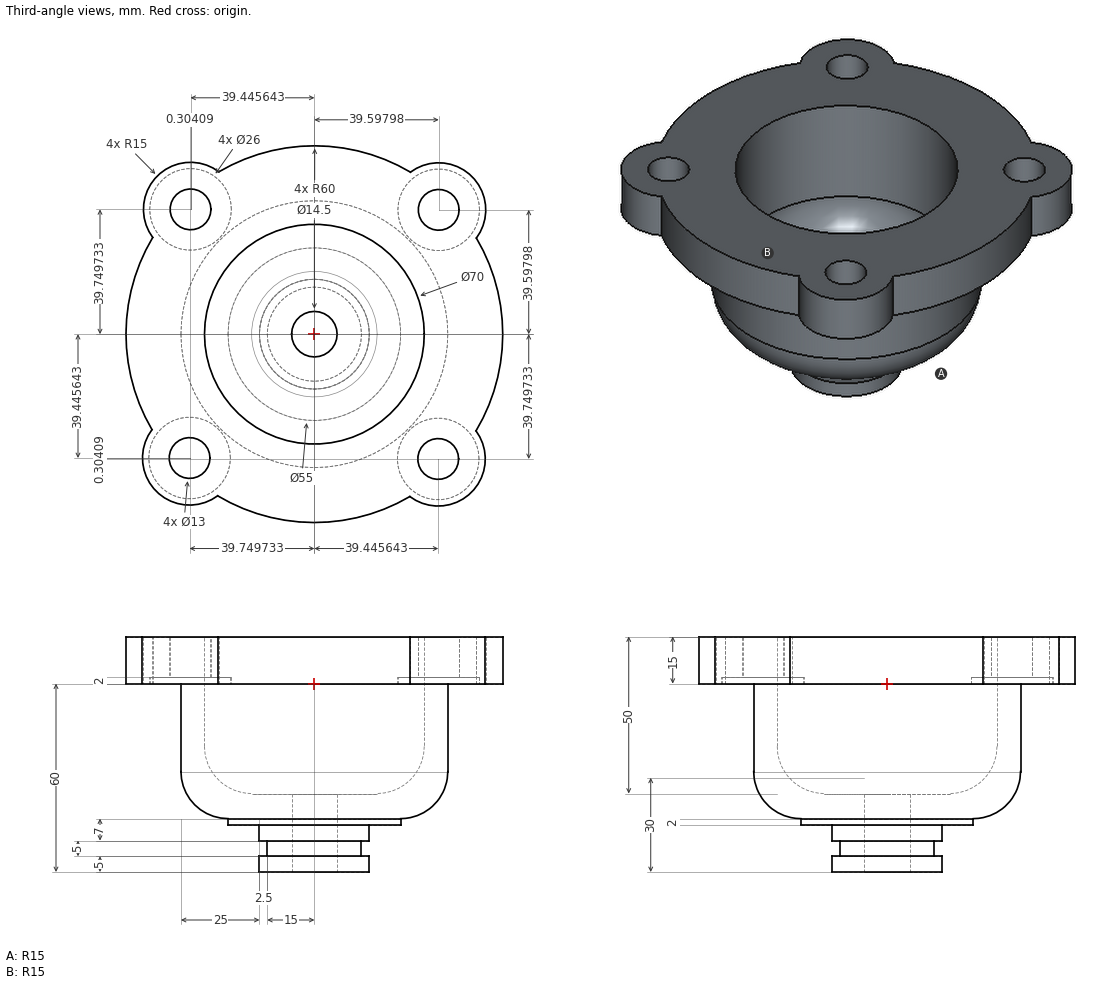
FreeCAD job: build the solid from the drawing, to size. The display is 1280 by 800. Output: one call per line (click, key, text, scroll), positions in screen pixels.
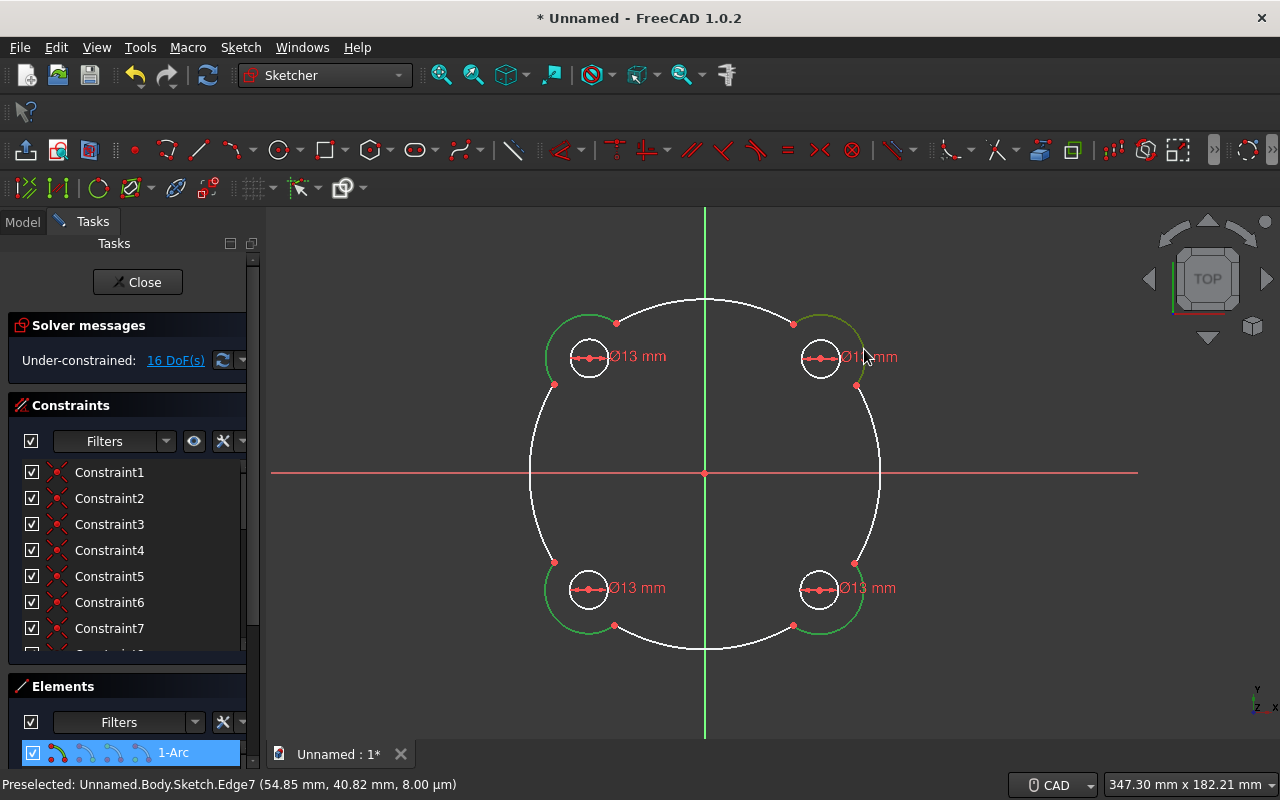
click(788, 150)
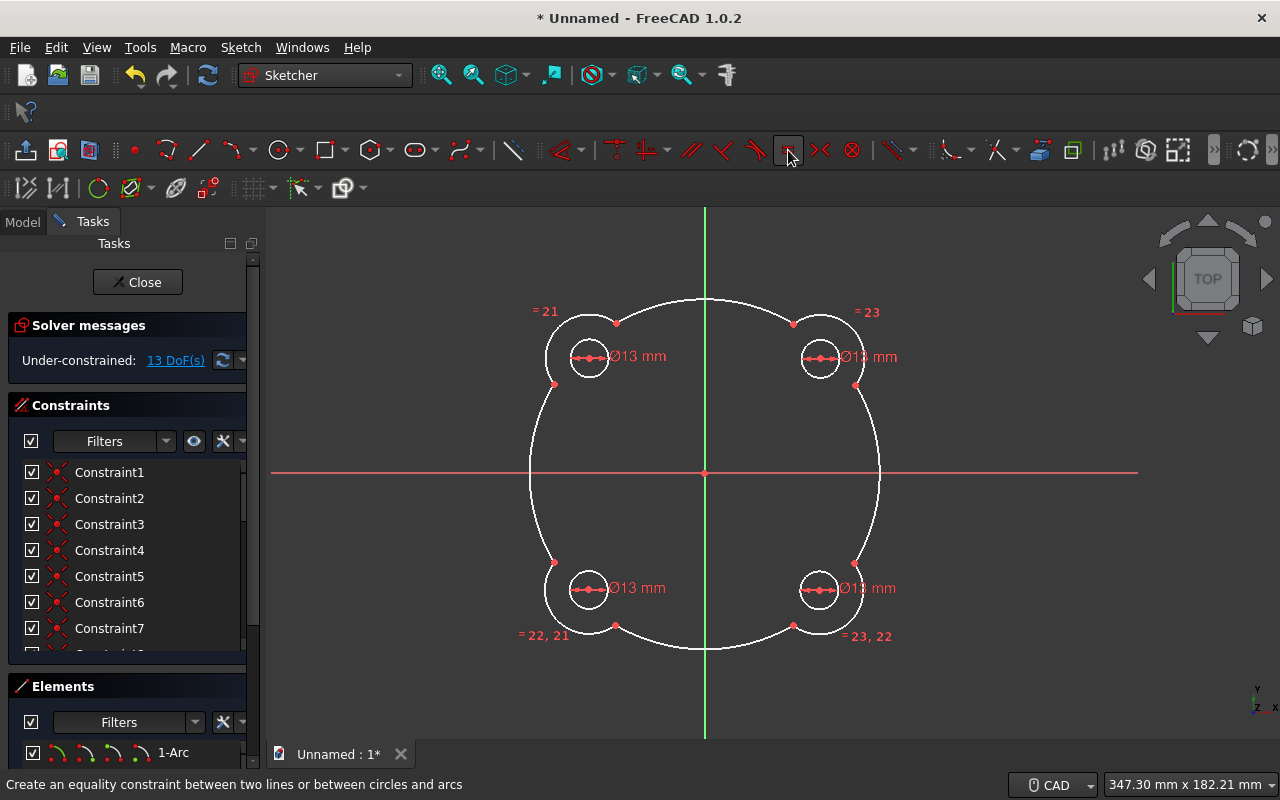
click(534, 436)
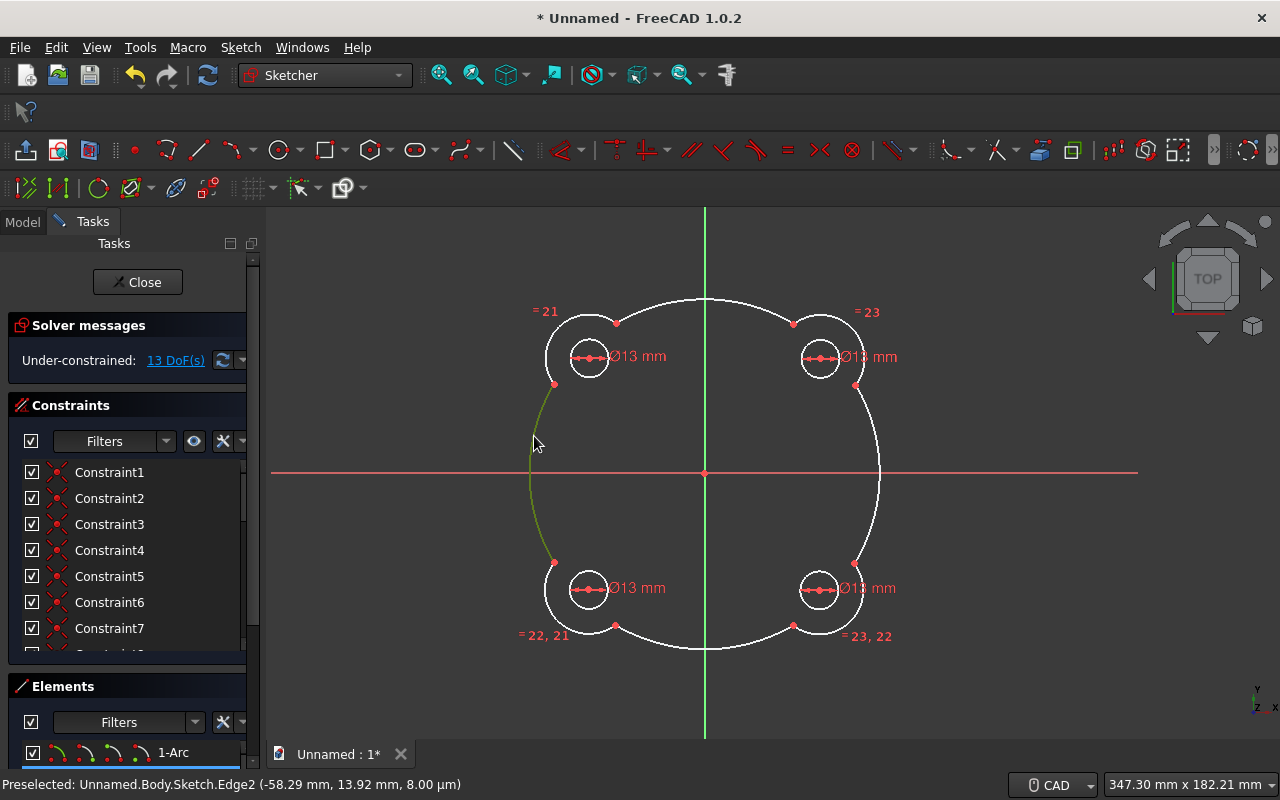
click(667, 645)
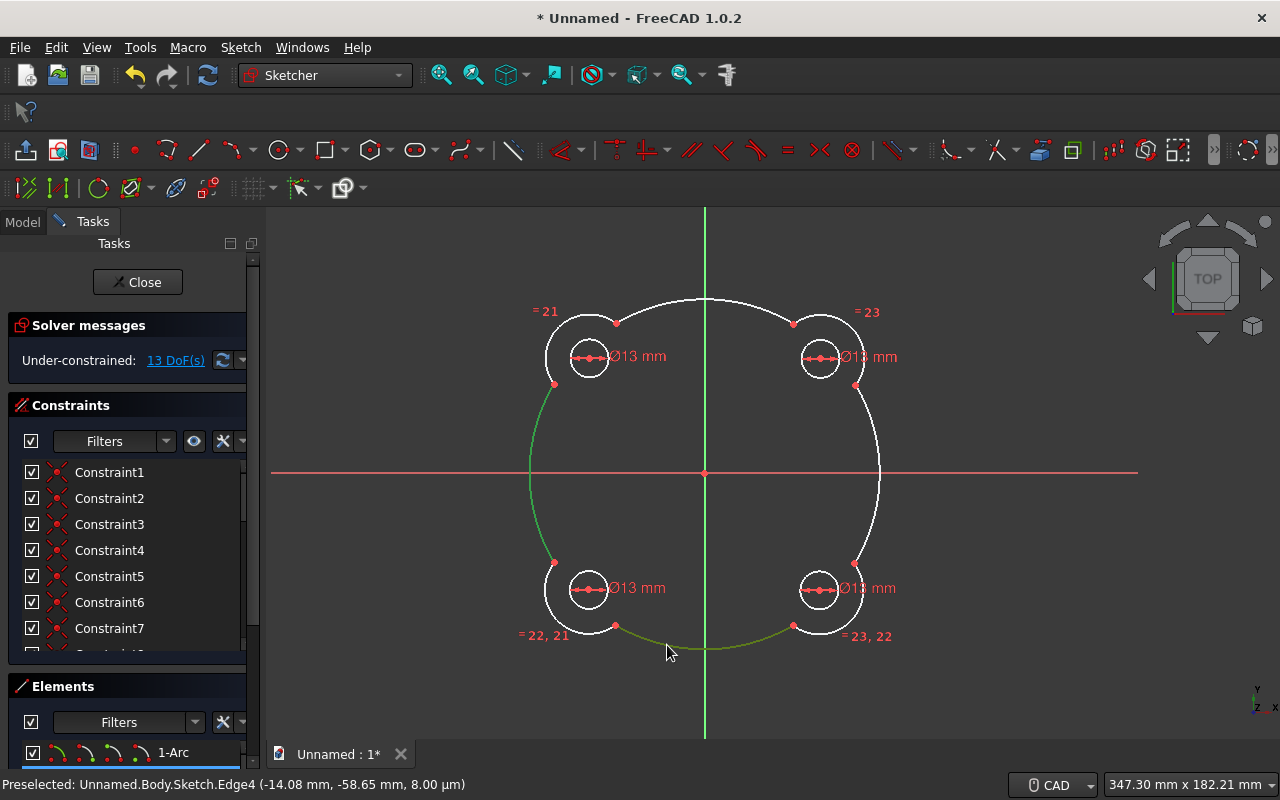
click(875, 512)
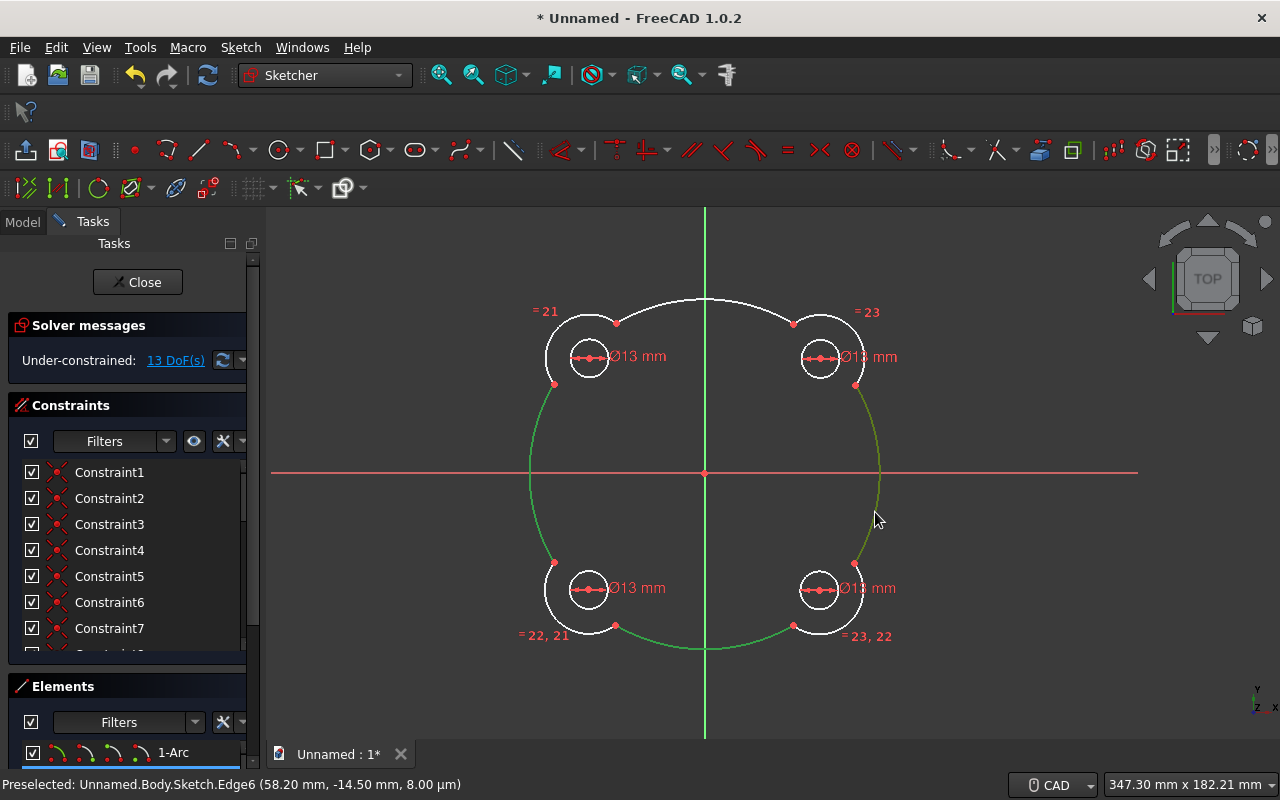
click(742, 303)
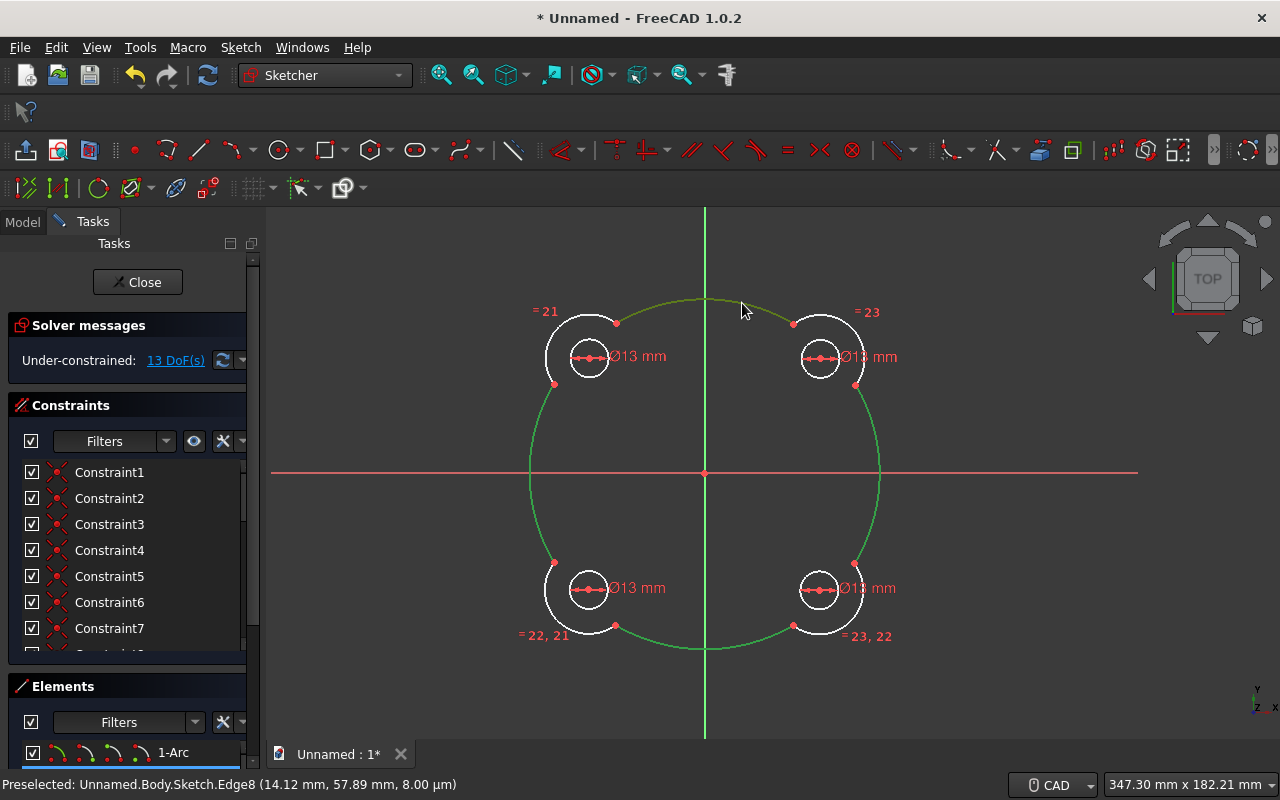
click(788, 150)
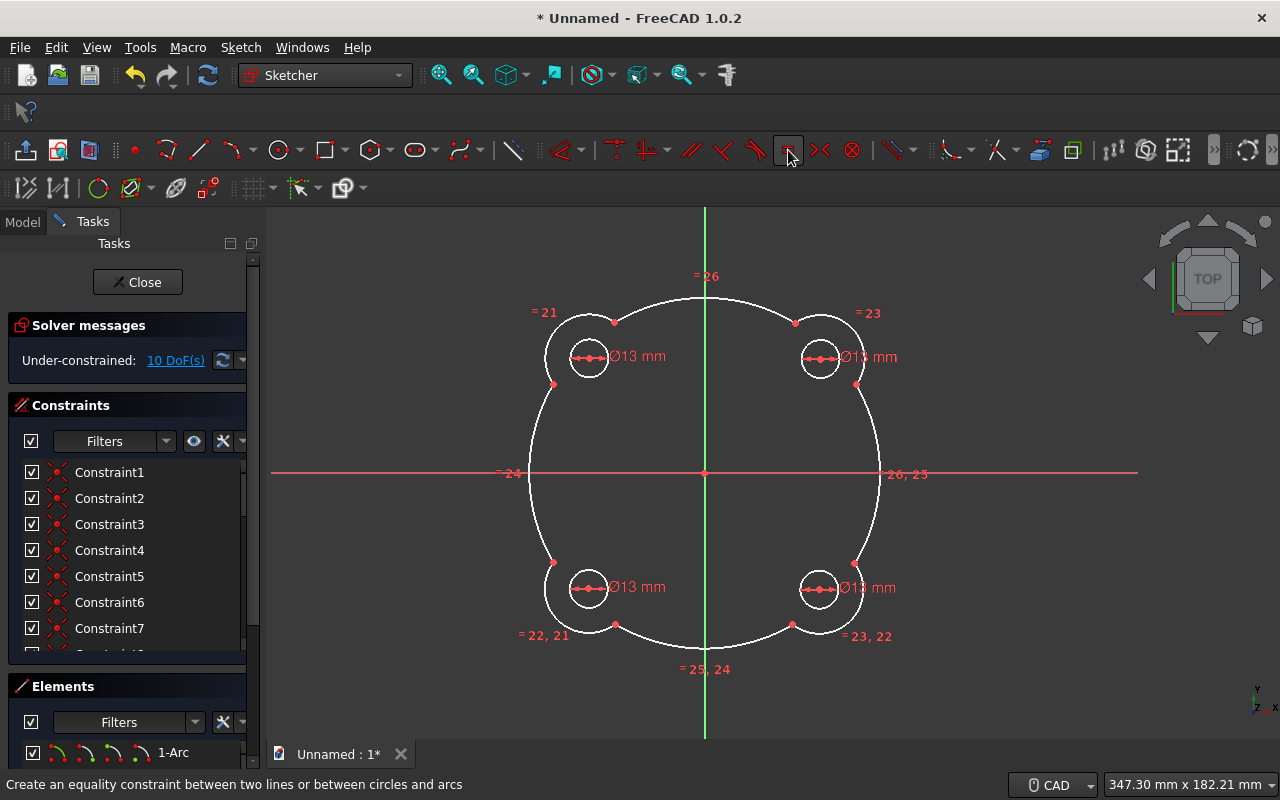
click(580, 316)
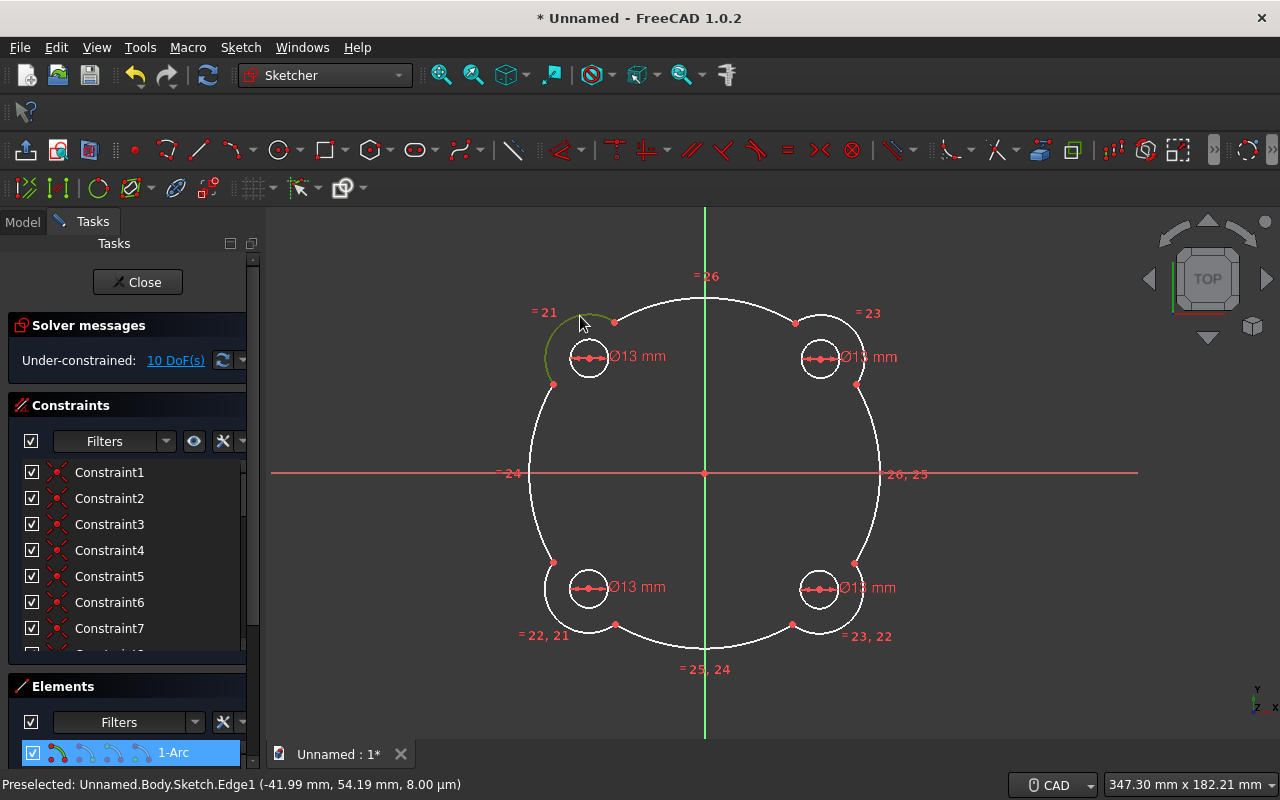
click(584, 150)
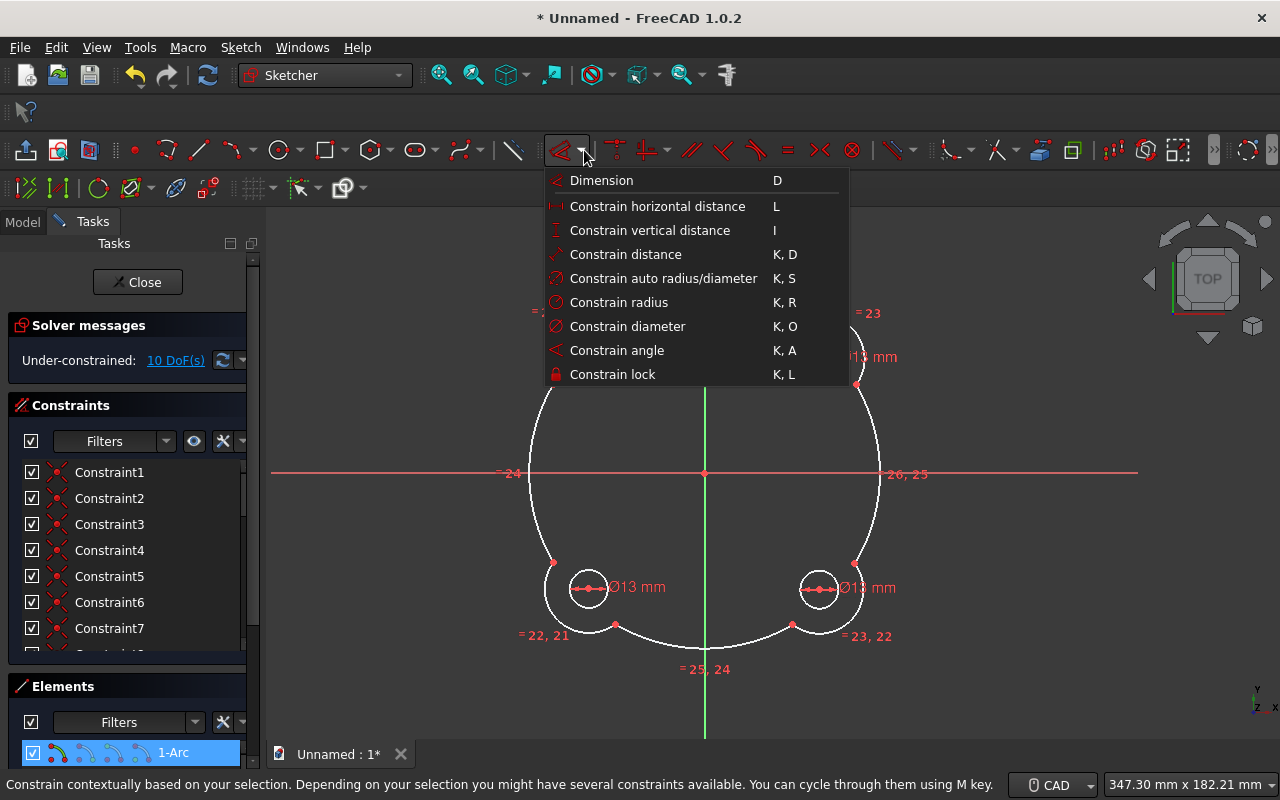
click(697, 302)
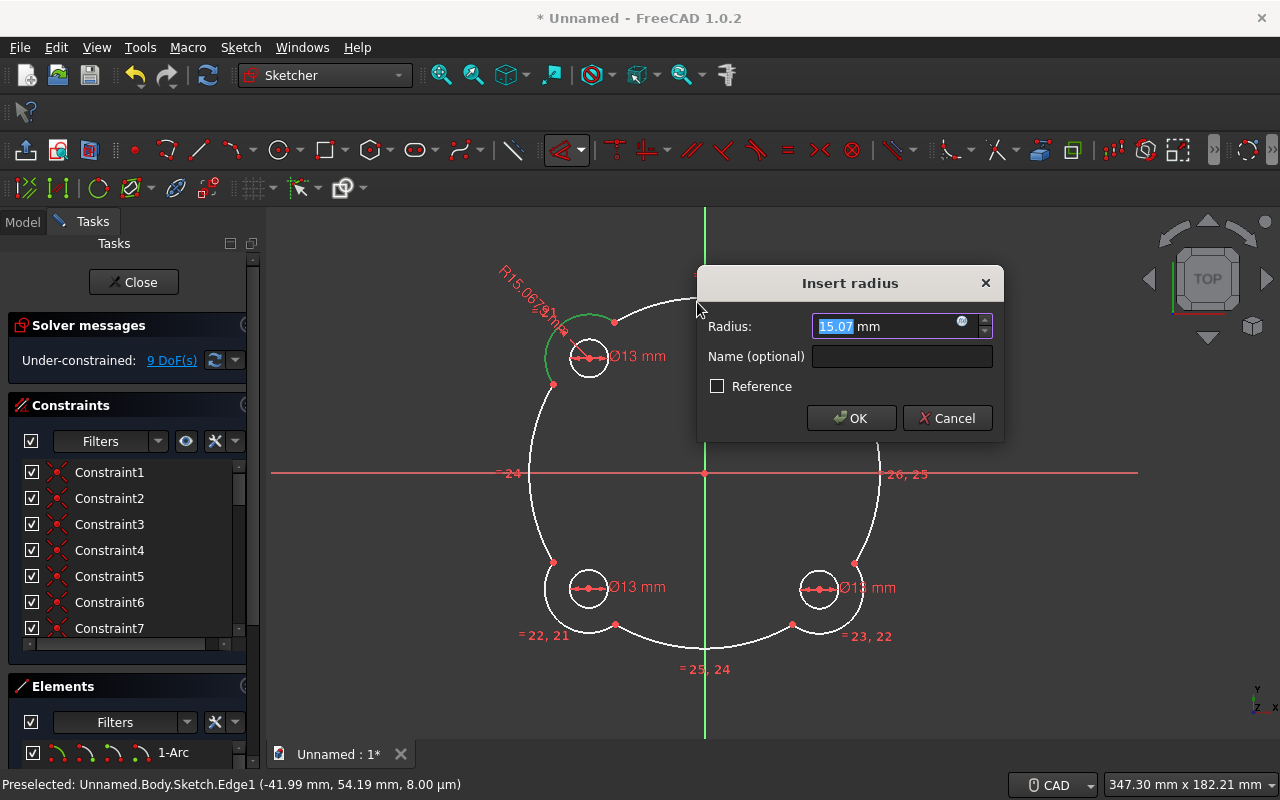
text(15)
key(Return)